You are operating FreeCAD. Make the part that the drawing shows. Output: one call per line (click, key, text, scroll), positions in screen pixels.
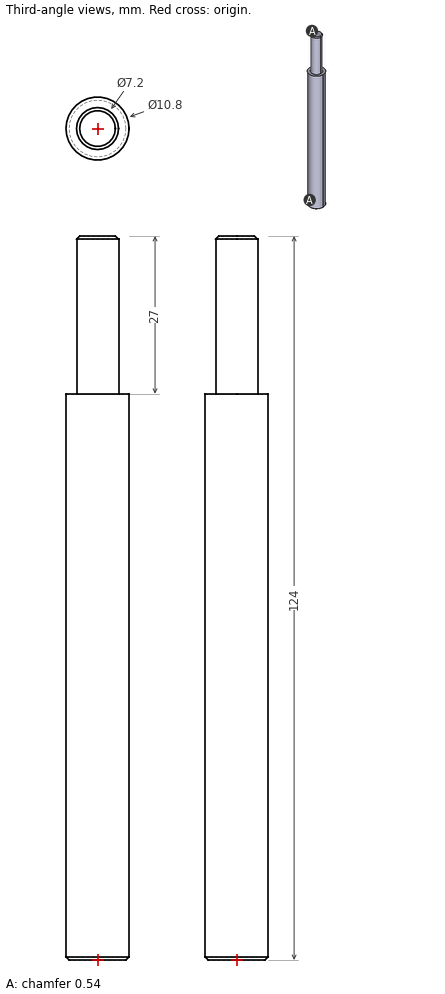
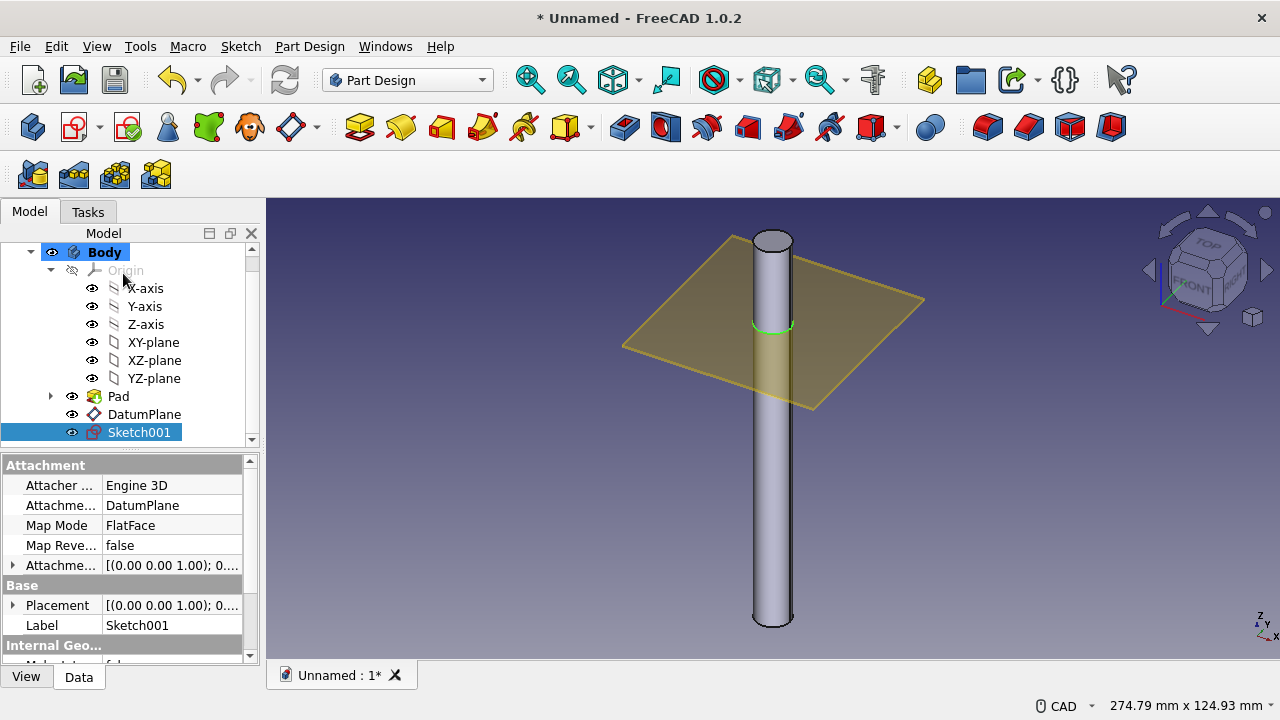
click(625, 128)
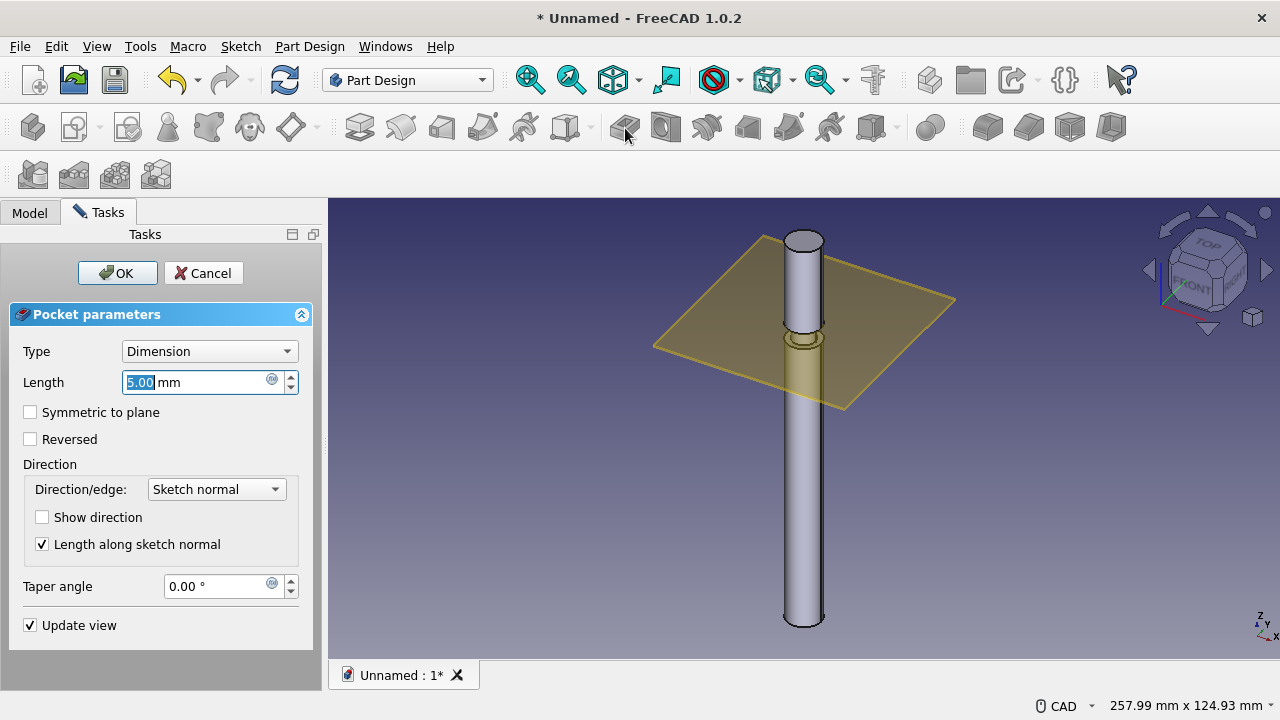
text(27)
key(Tab)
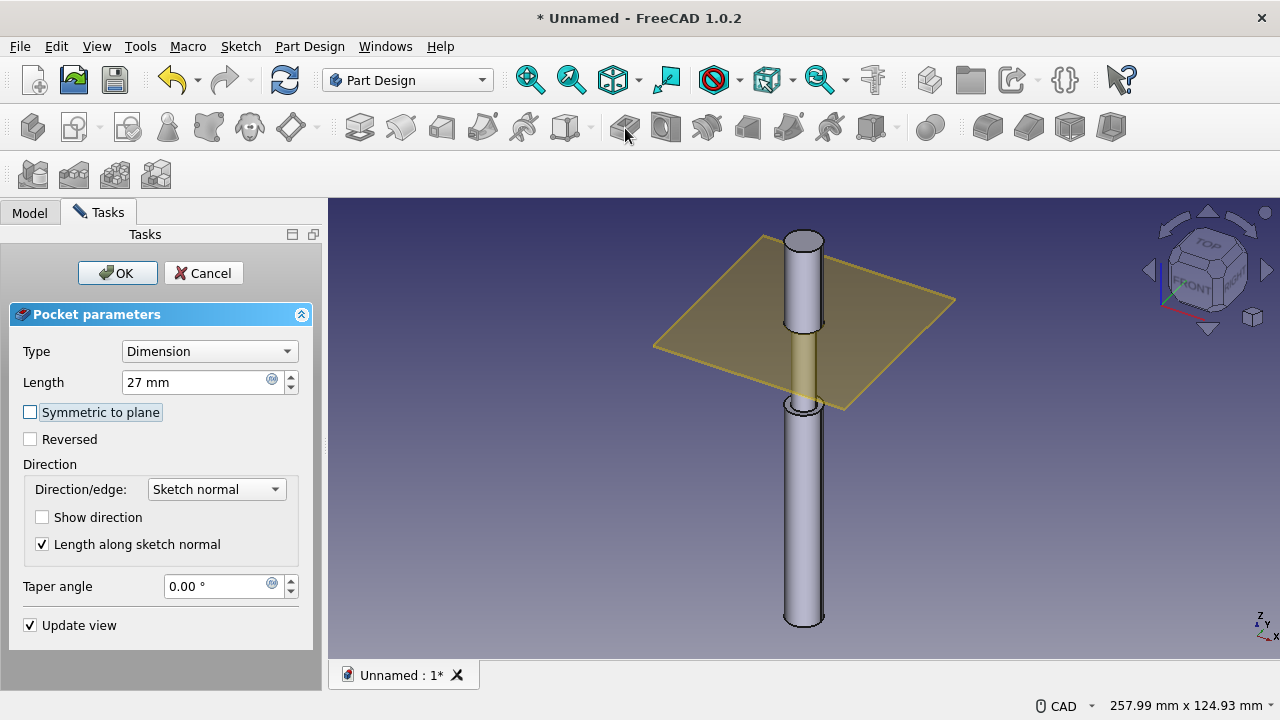
click(31, 439)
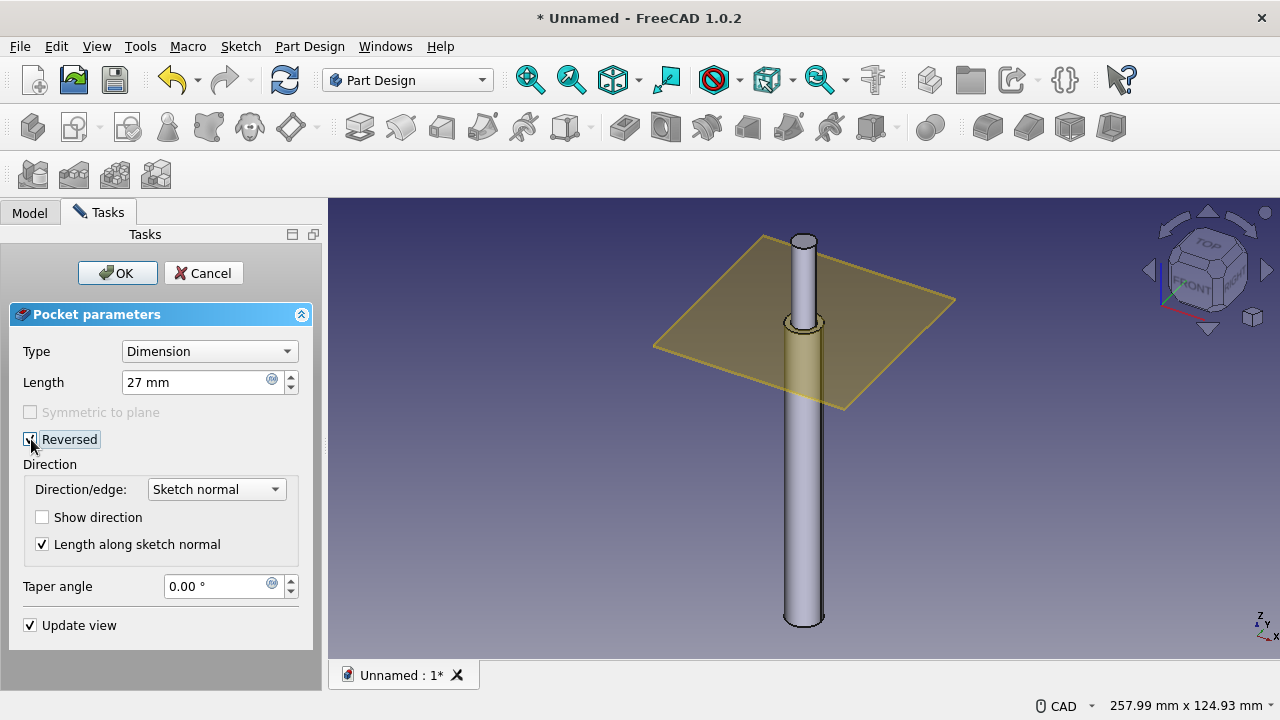
click(118, 273)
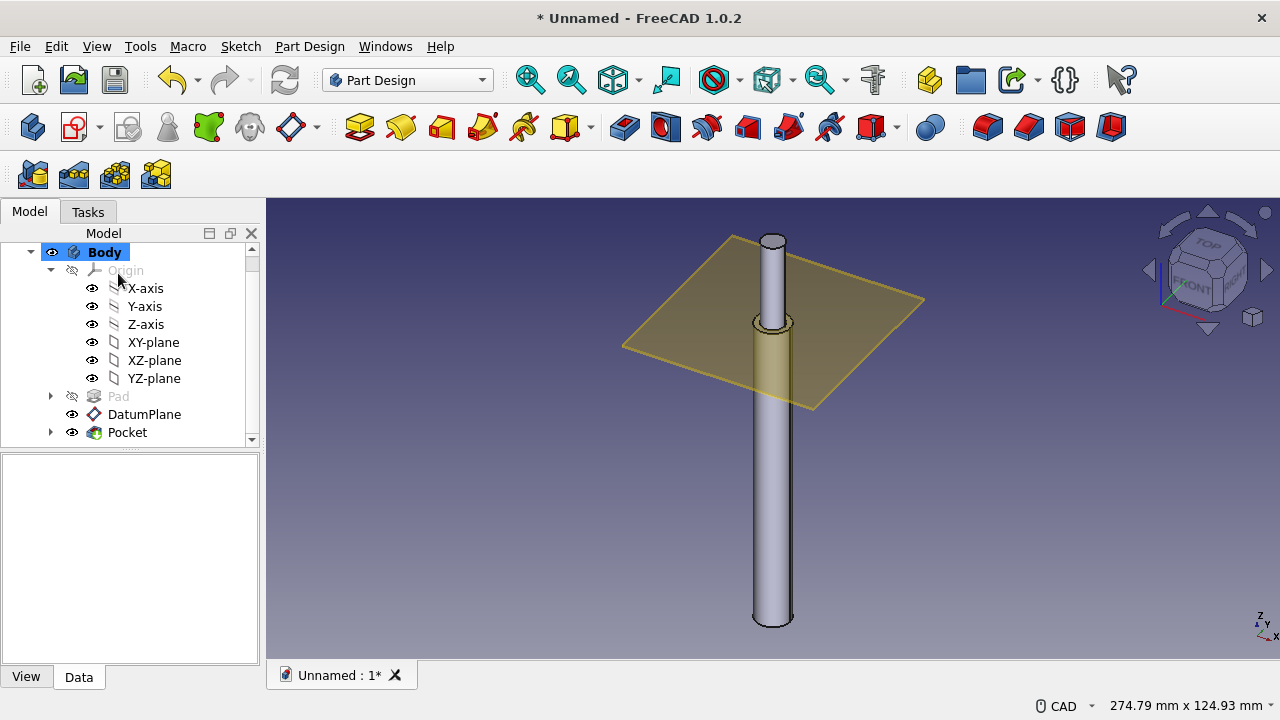
click(117, 414)
key(space)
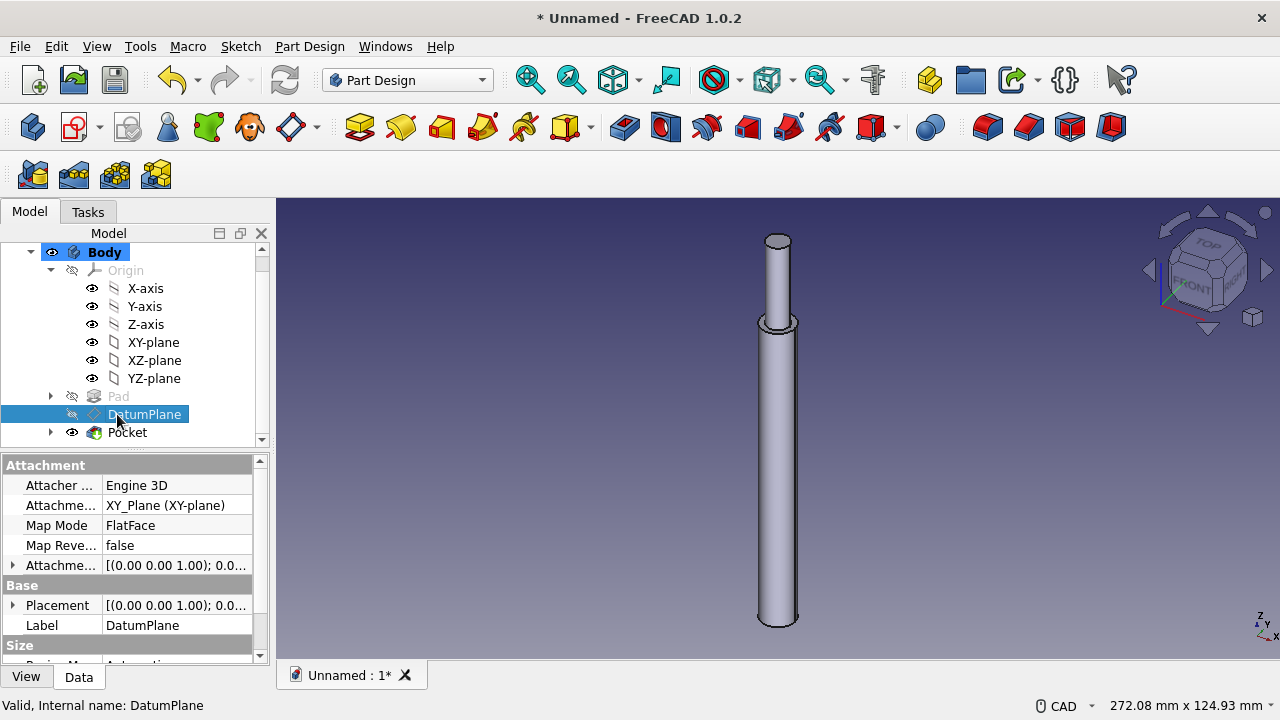
click(763, 623)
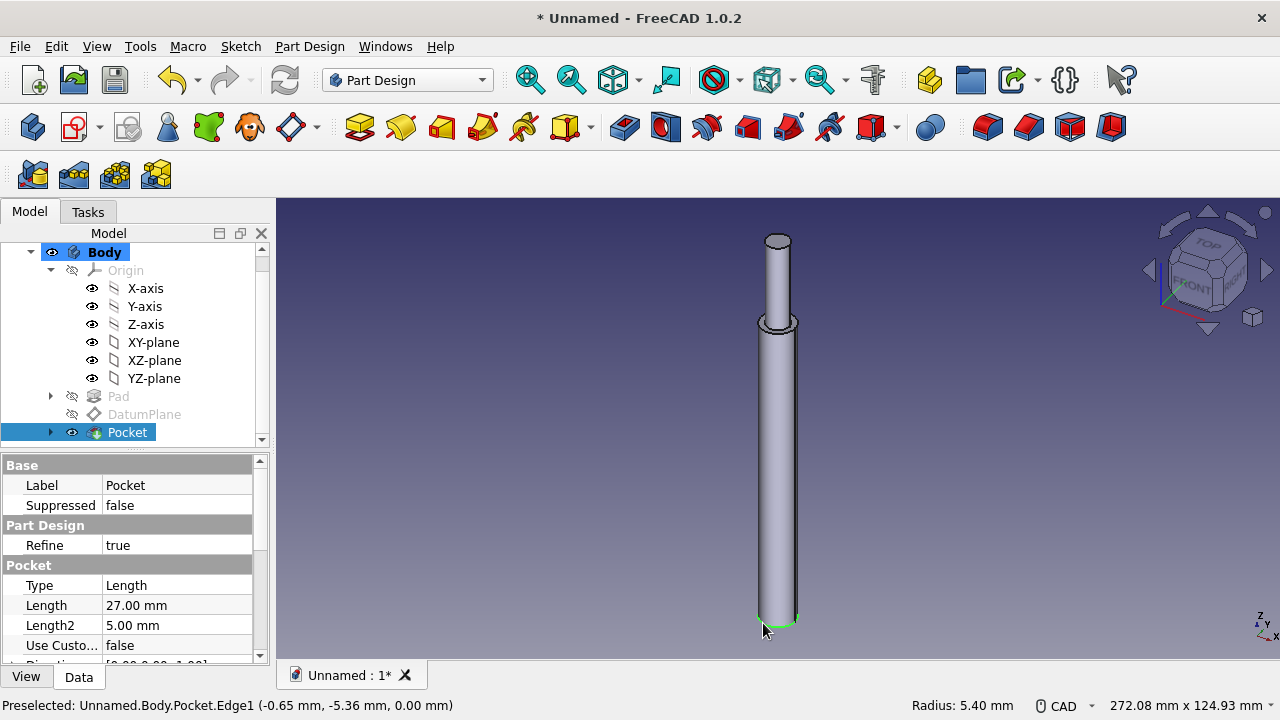
click(766, 236, ctrl)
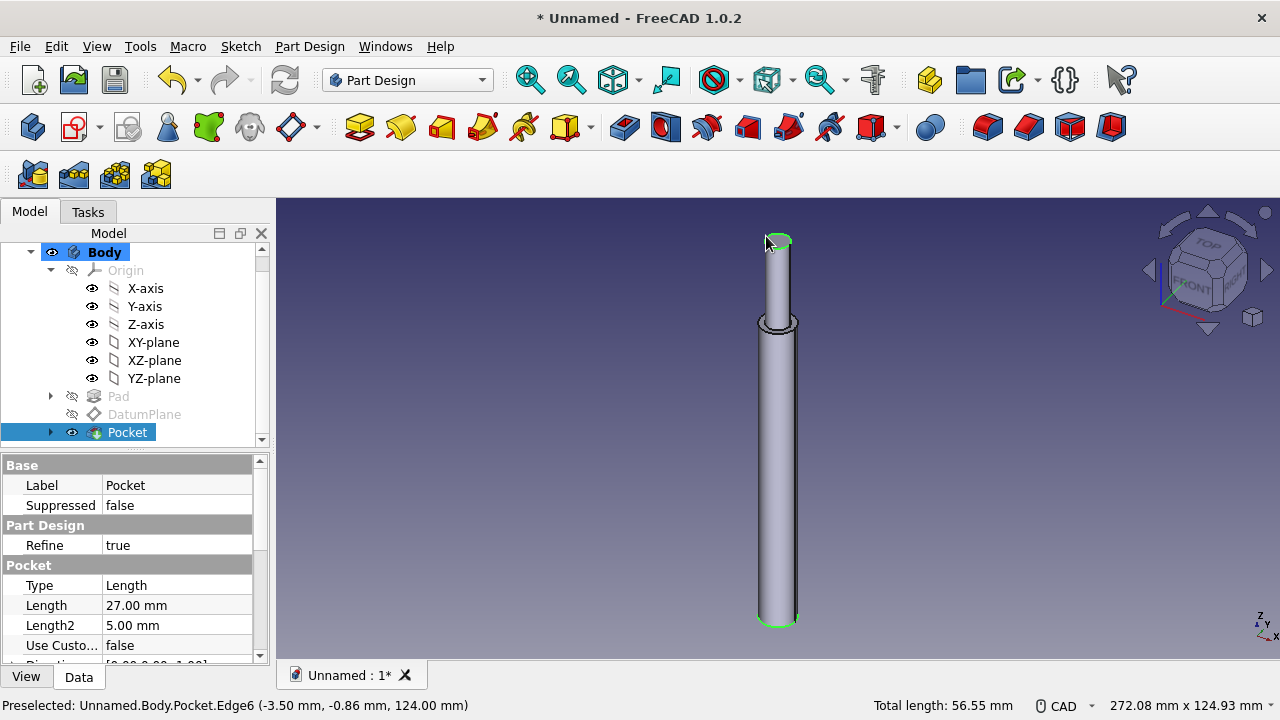
click(1029, 128)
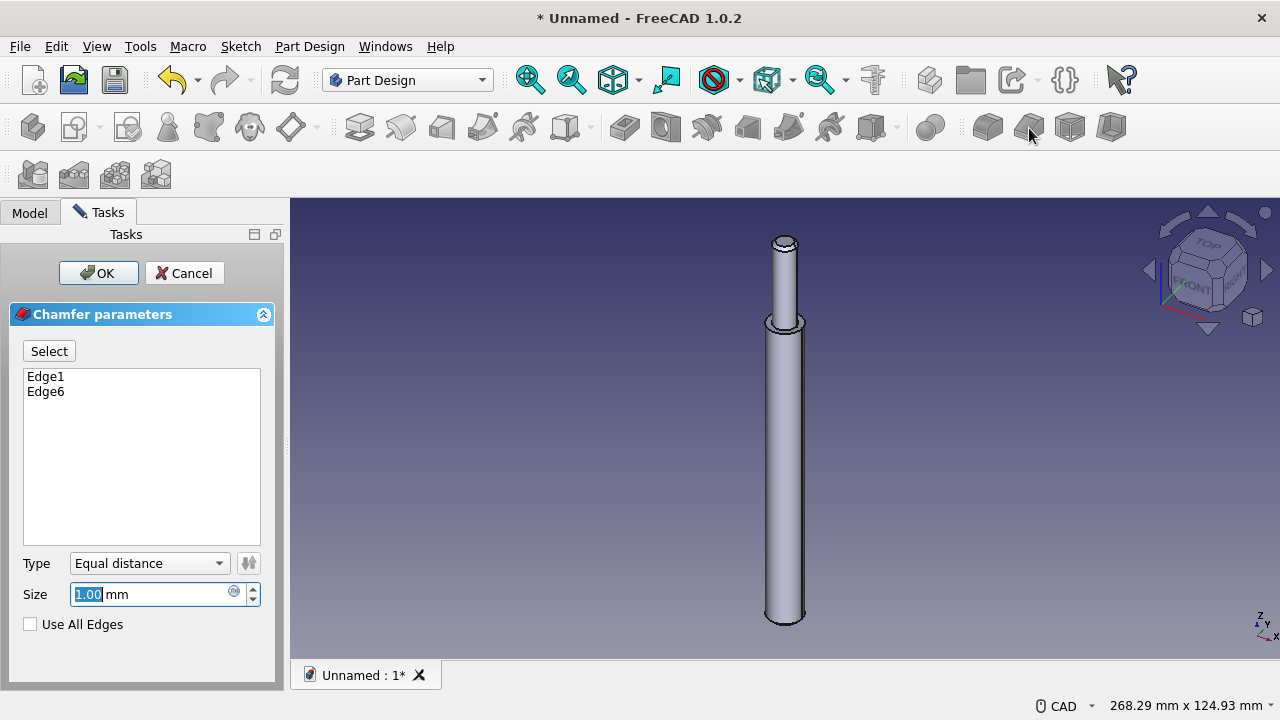
text(0.54)
key(Tab)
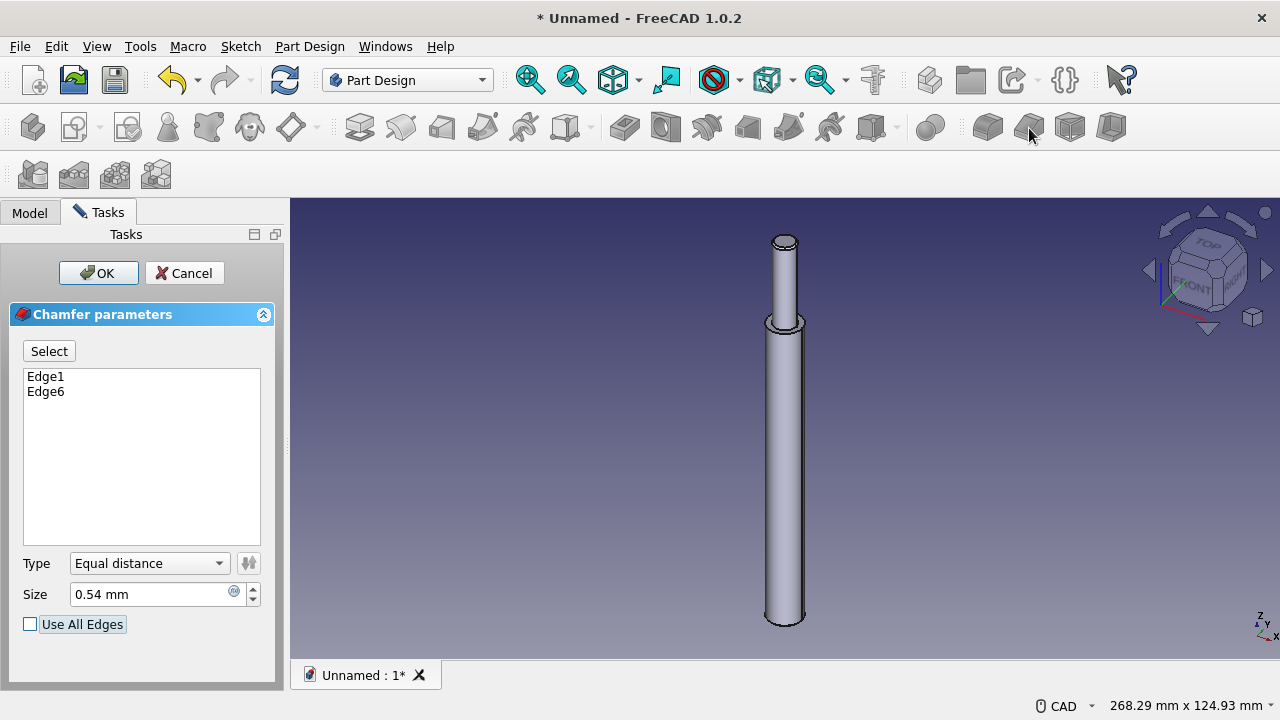
click(99, 273)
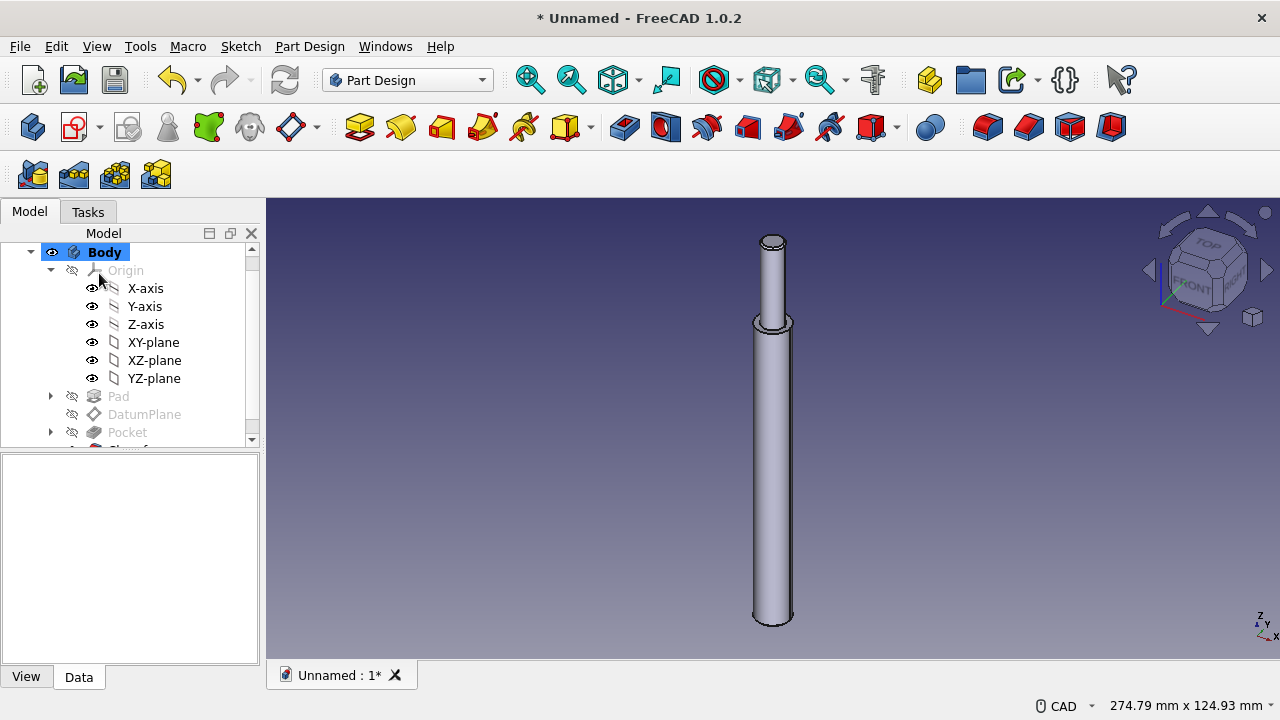
key(0)